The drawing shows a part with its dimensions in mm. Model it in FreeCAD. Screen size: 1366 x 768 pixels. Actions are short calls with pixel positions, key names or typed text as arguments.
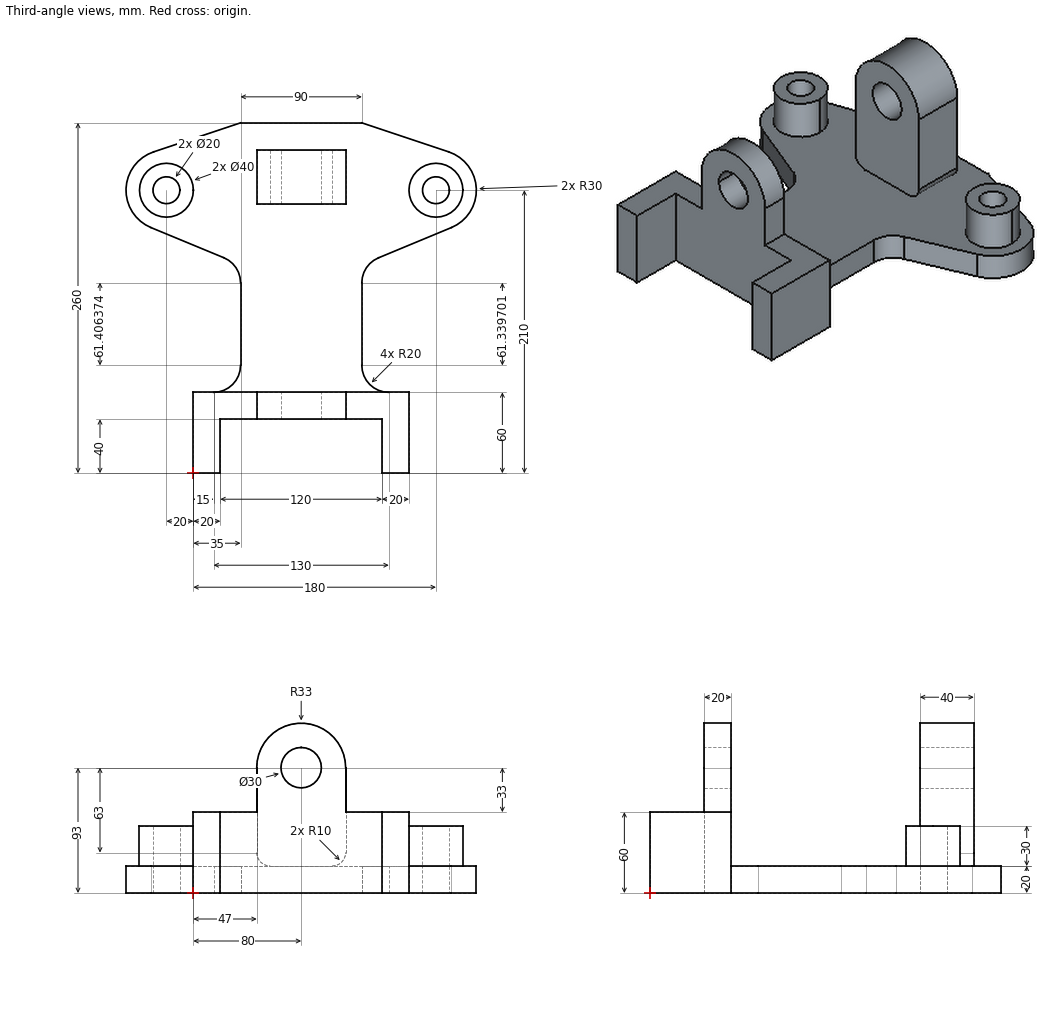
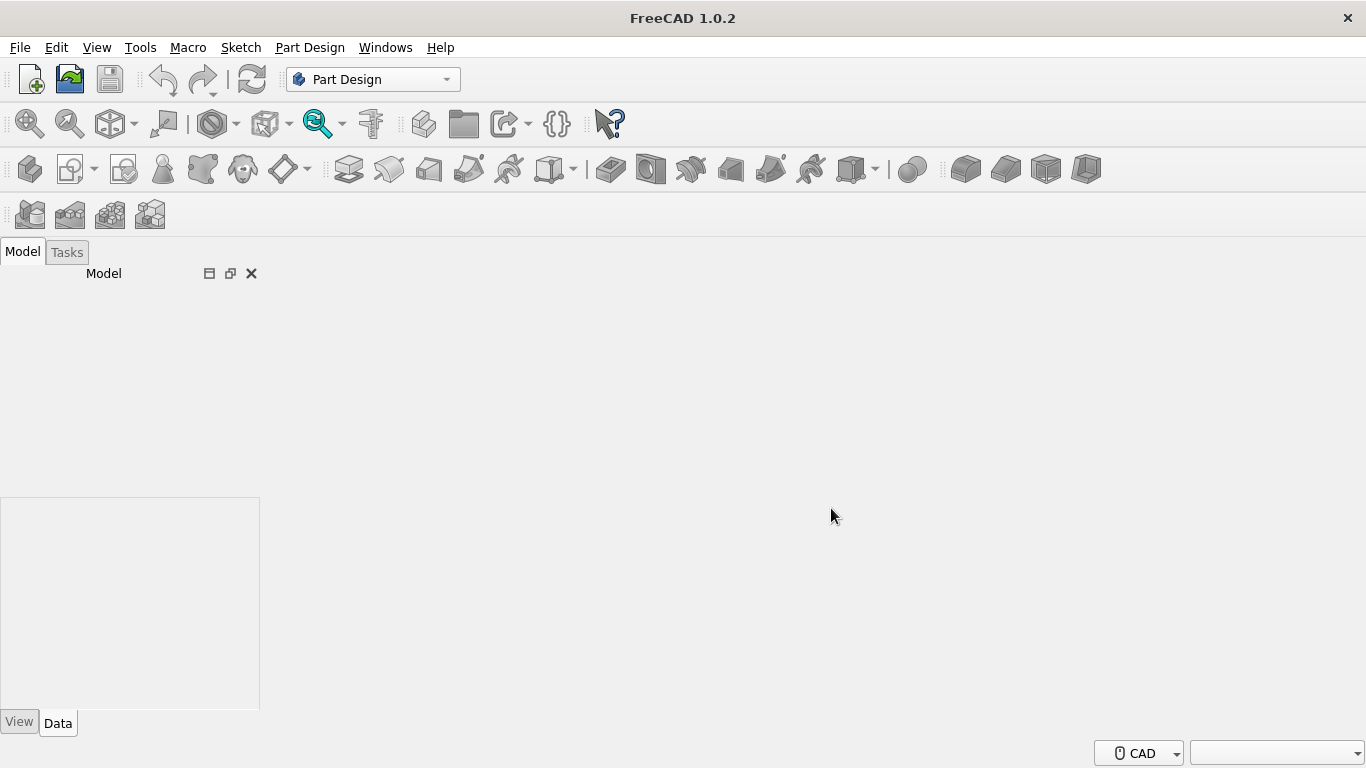
click(30, 80)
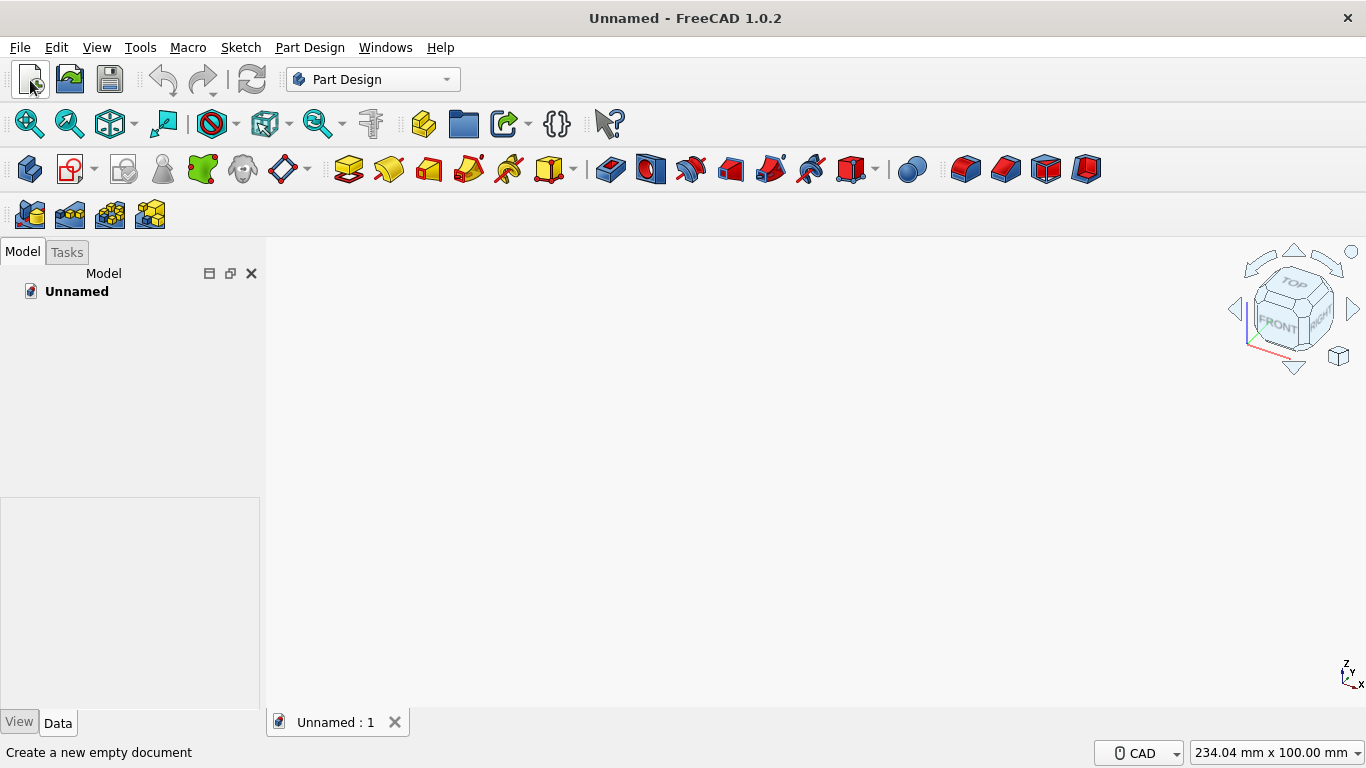
click(70, 170)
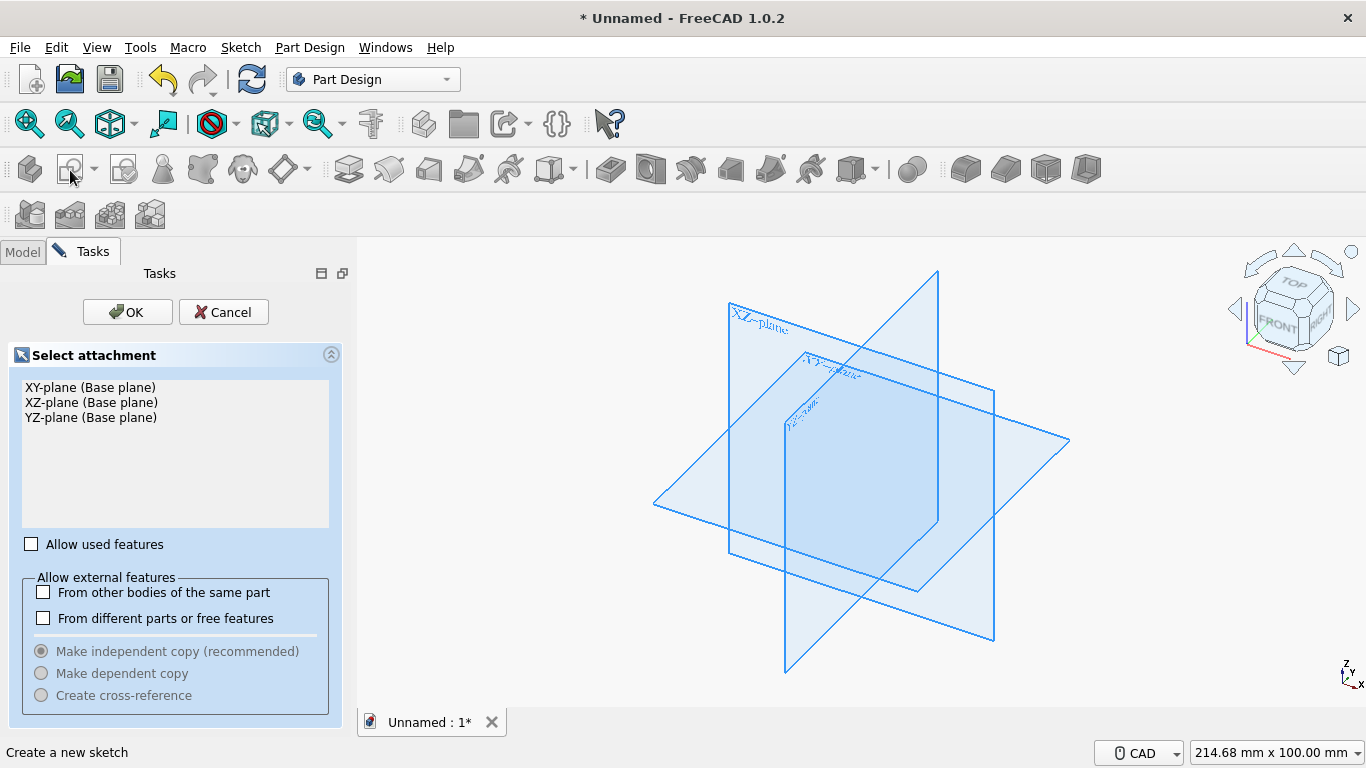
click(82, 388)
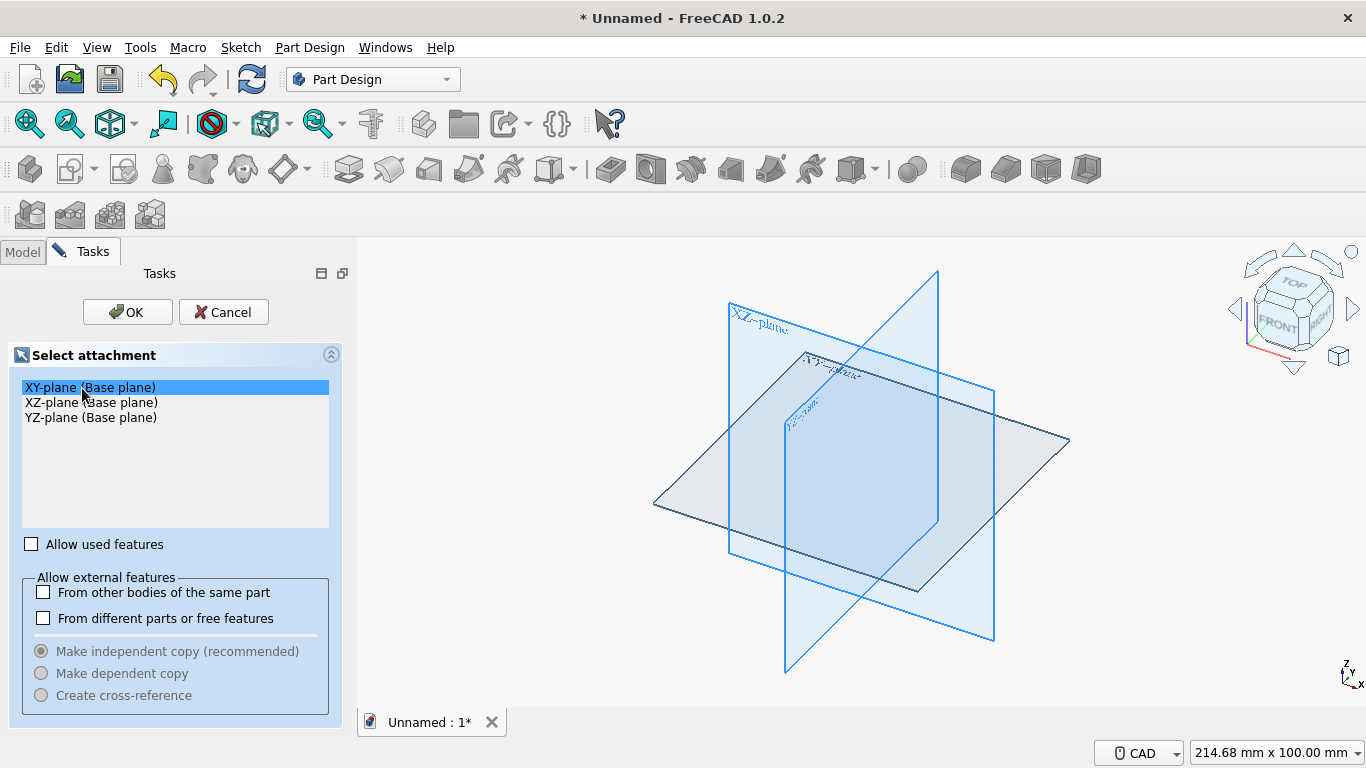
click(128, 312)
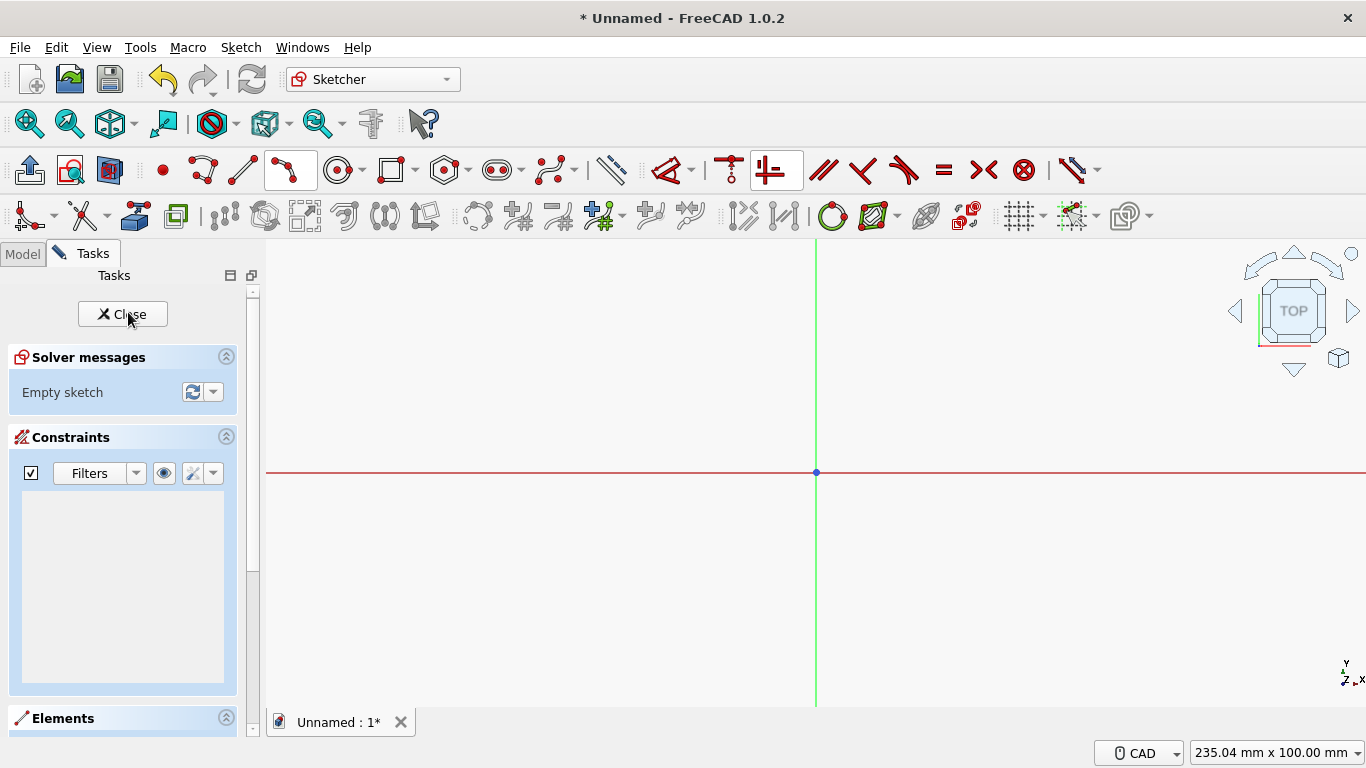
scroll(294, 679, down, 2)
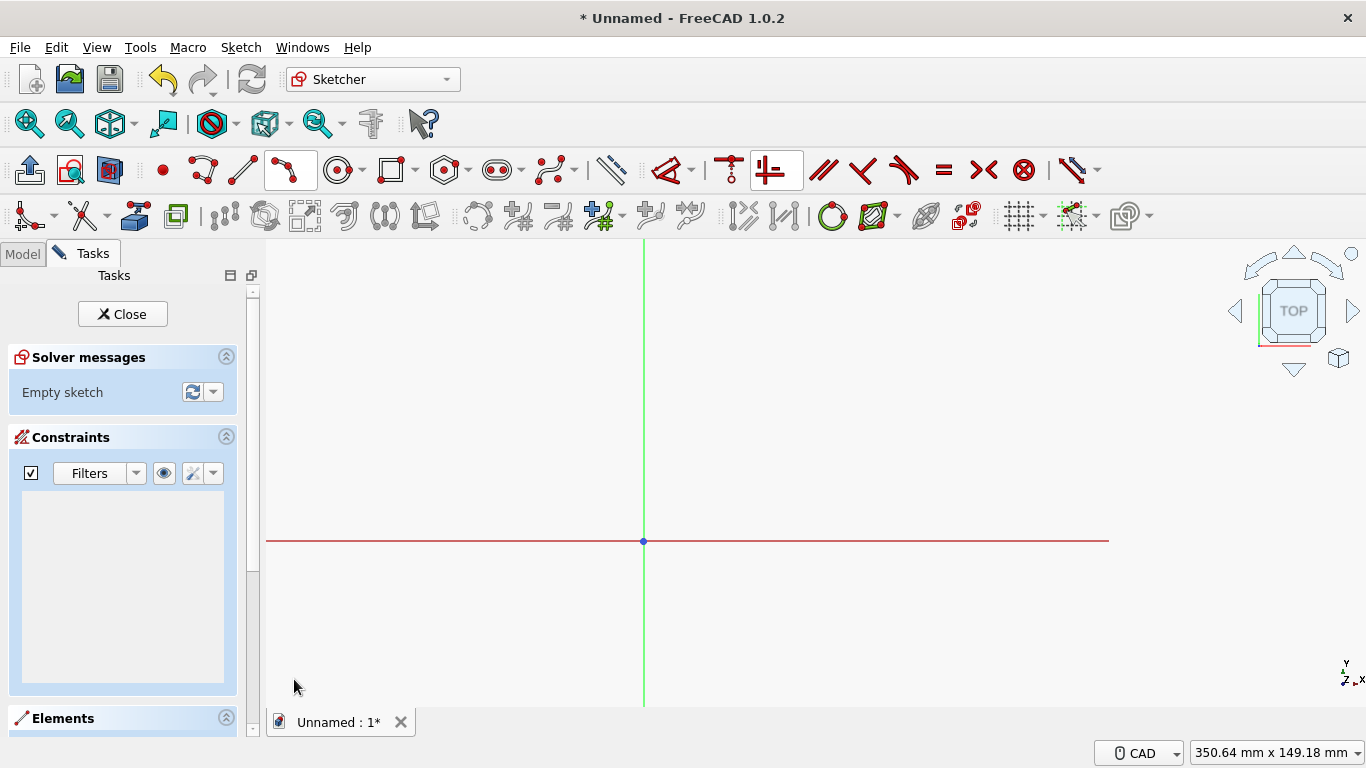
click(204, 170)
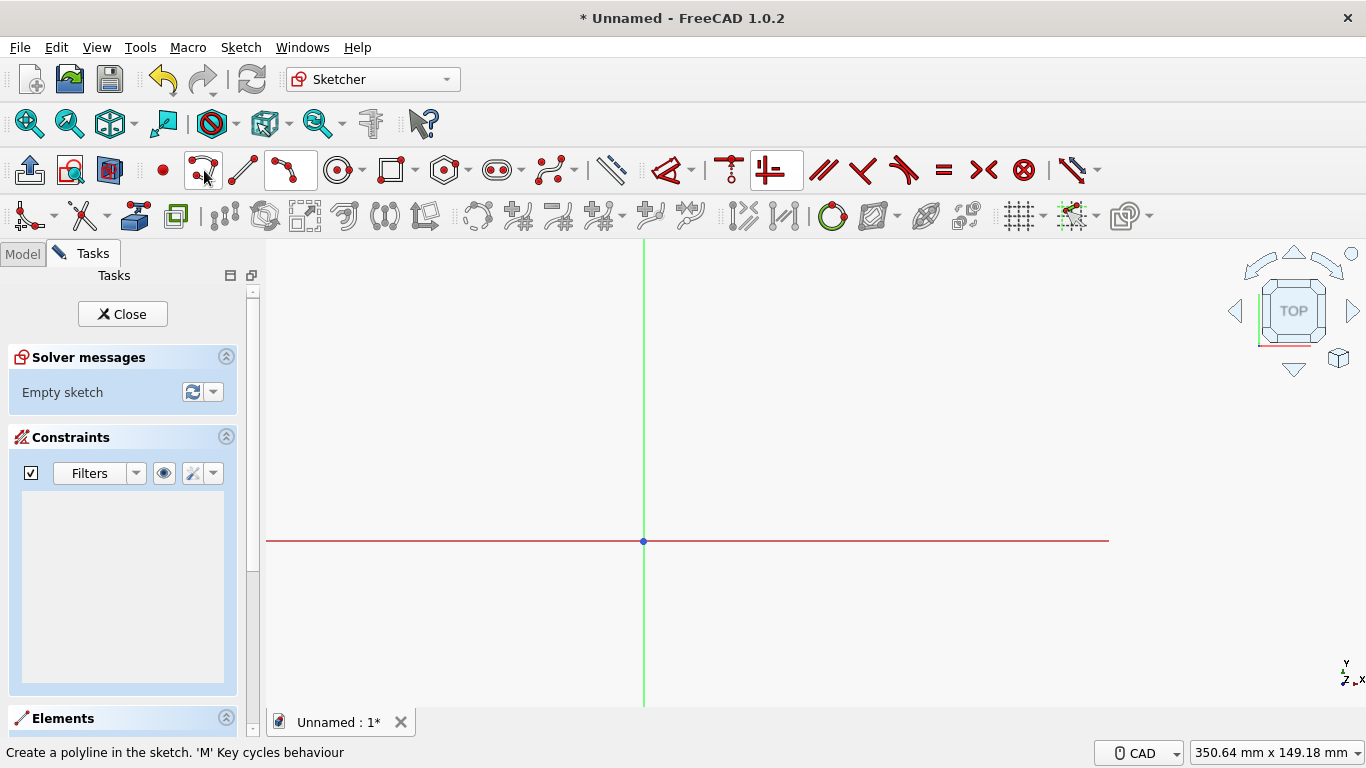
click(644, 541)
click(707, 532)
click(707, 416)
click(1083, 416)
click(1083, 541)
click(1146, 532)
click(1146, 353)
click(653, 353)
click(644, 541)
key(Escape)
key(Escape)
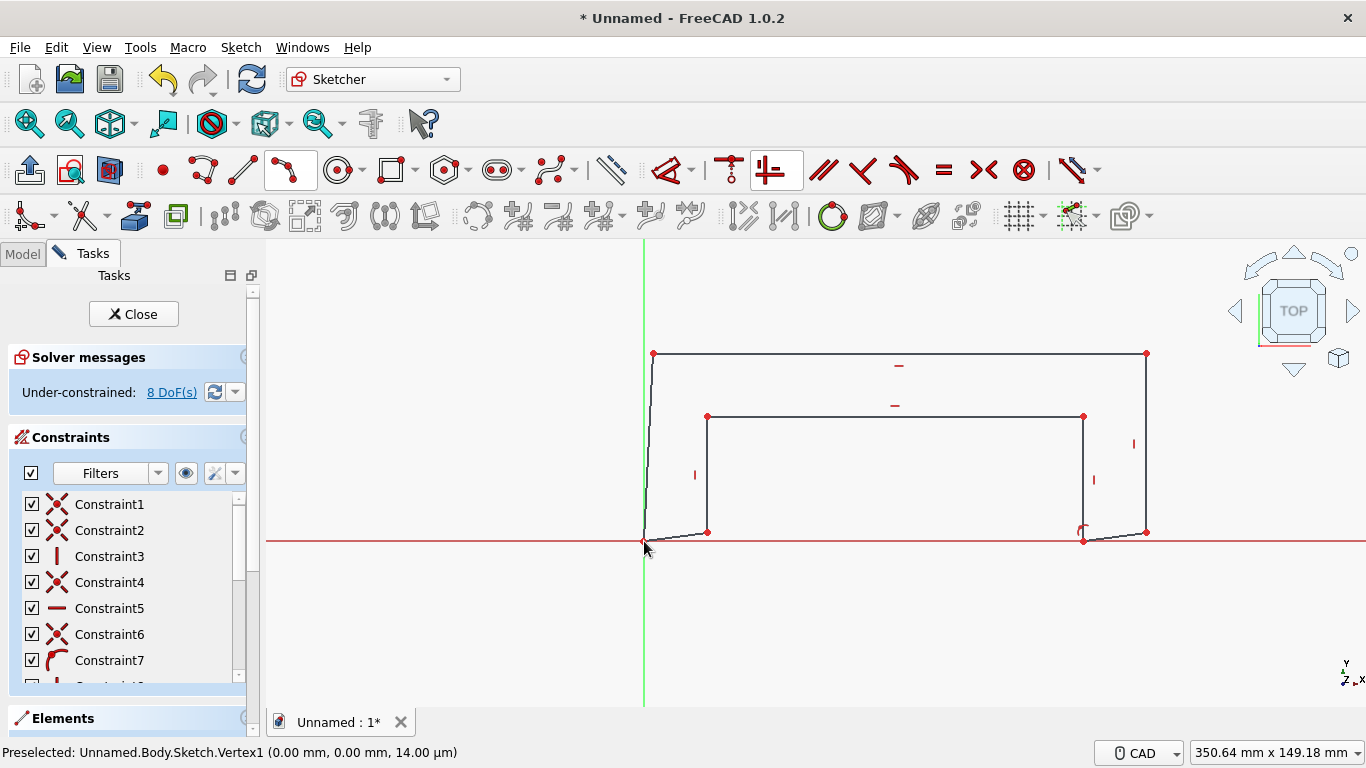
click(663, 539)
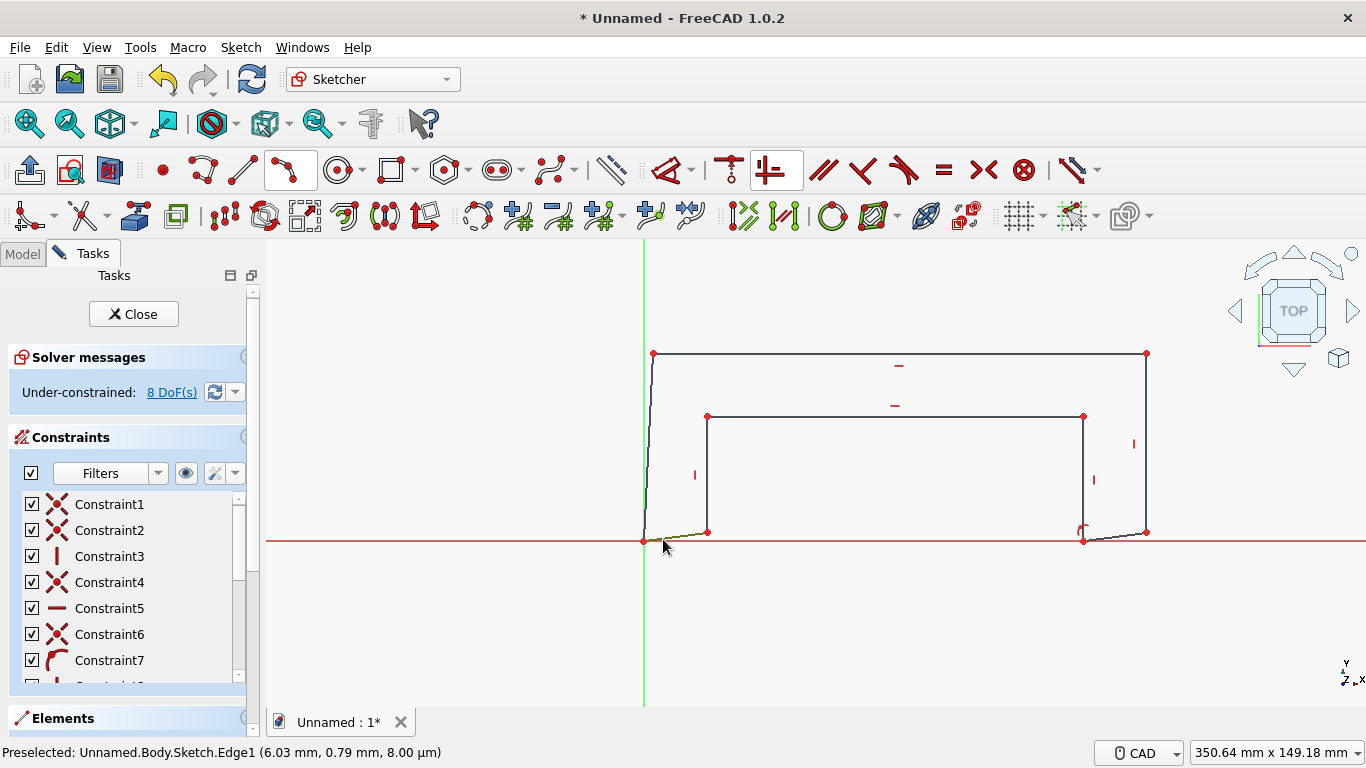
click(798, 170)